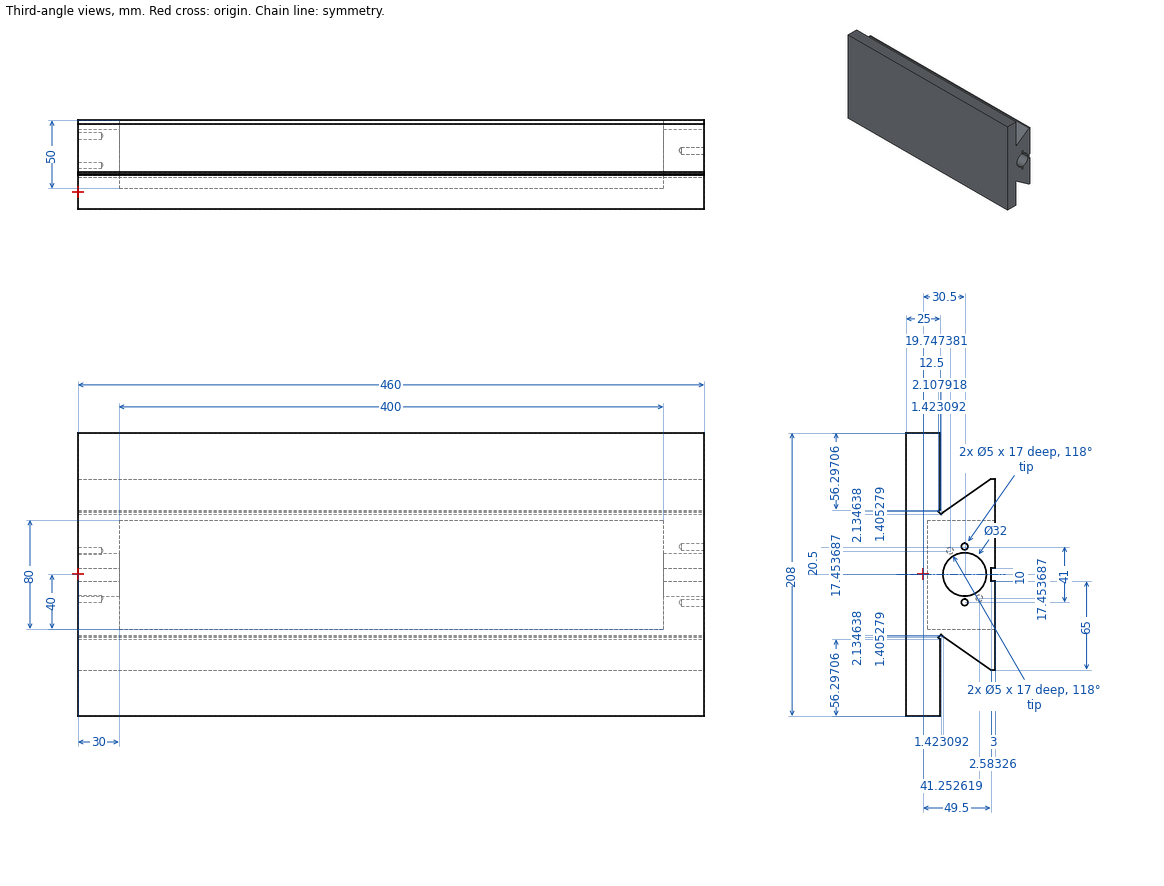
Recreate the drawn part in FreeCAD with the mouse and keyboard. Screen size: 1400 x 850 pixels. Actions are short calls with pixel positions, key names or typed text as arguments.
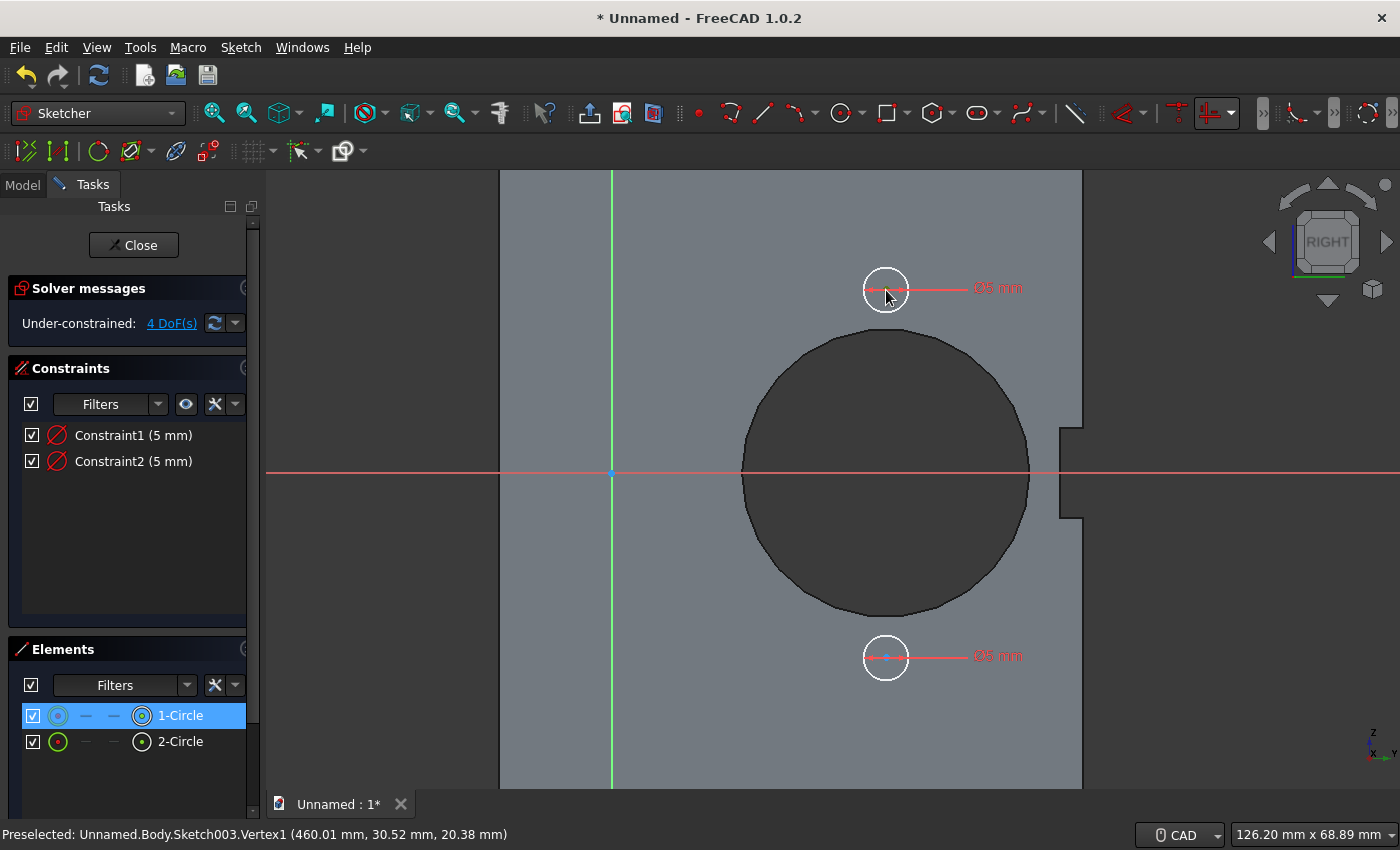
click(886, 658)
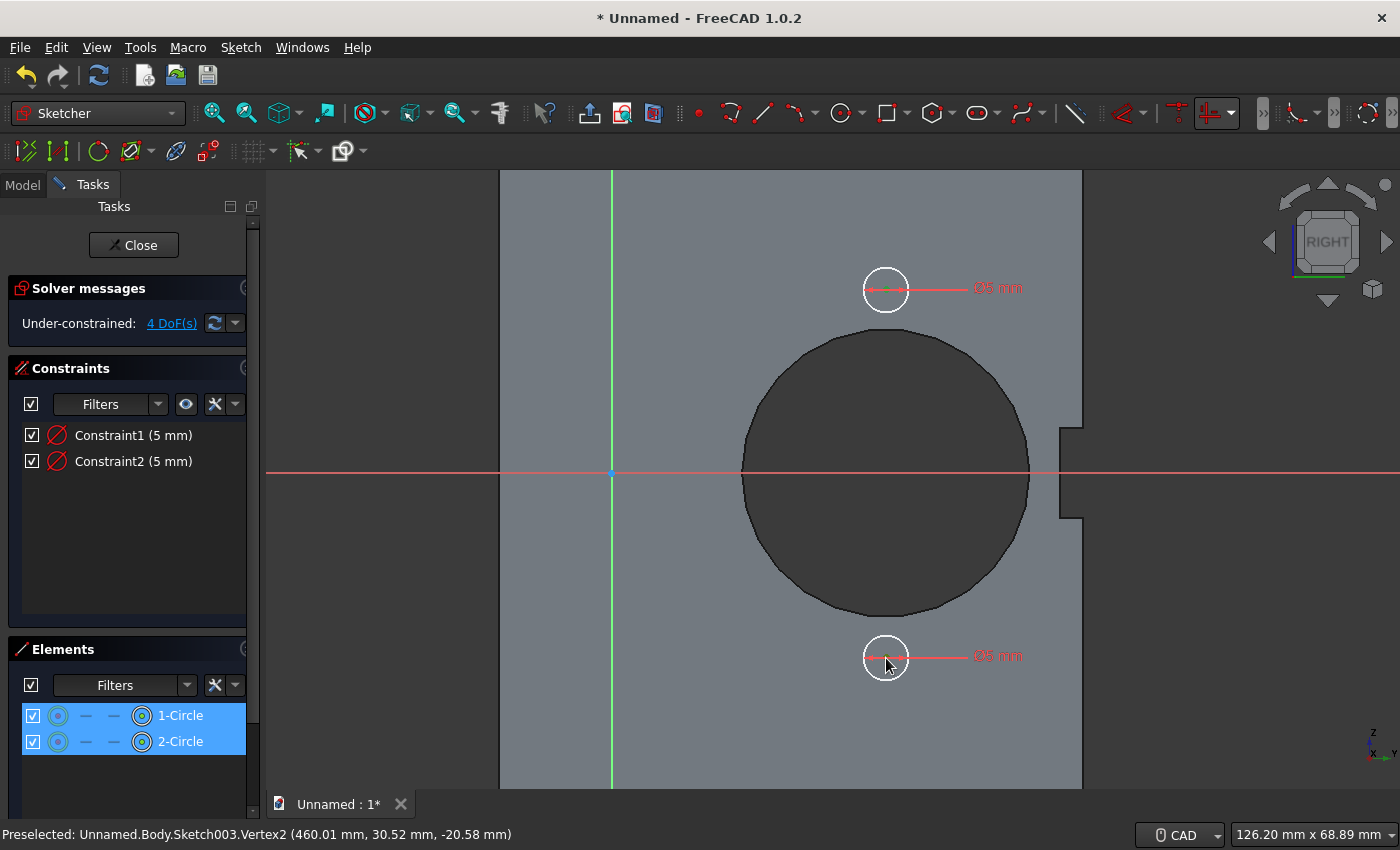
click(1234, 114)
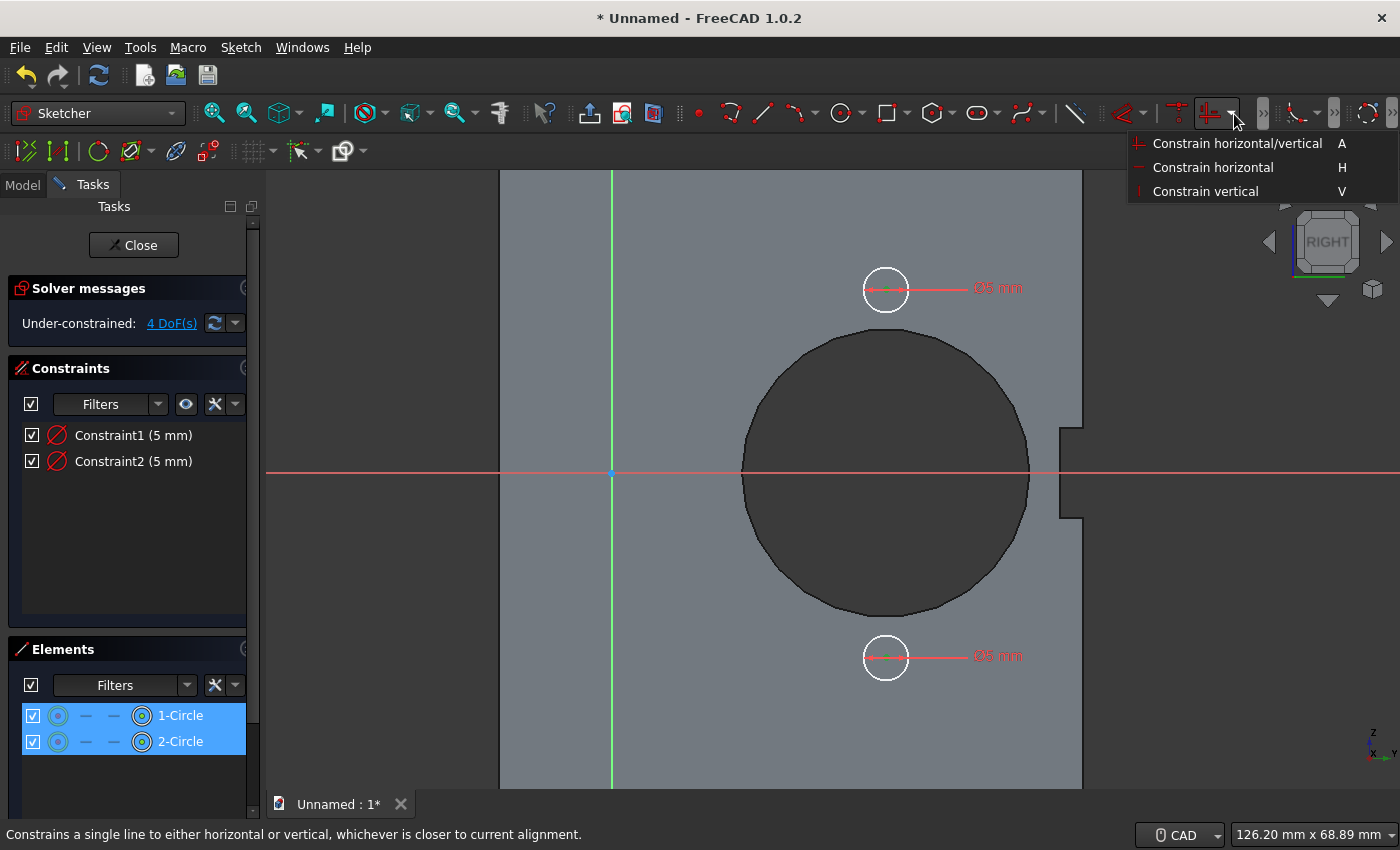
click(1263, 191)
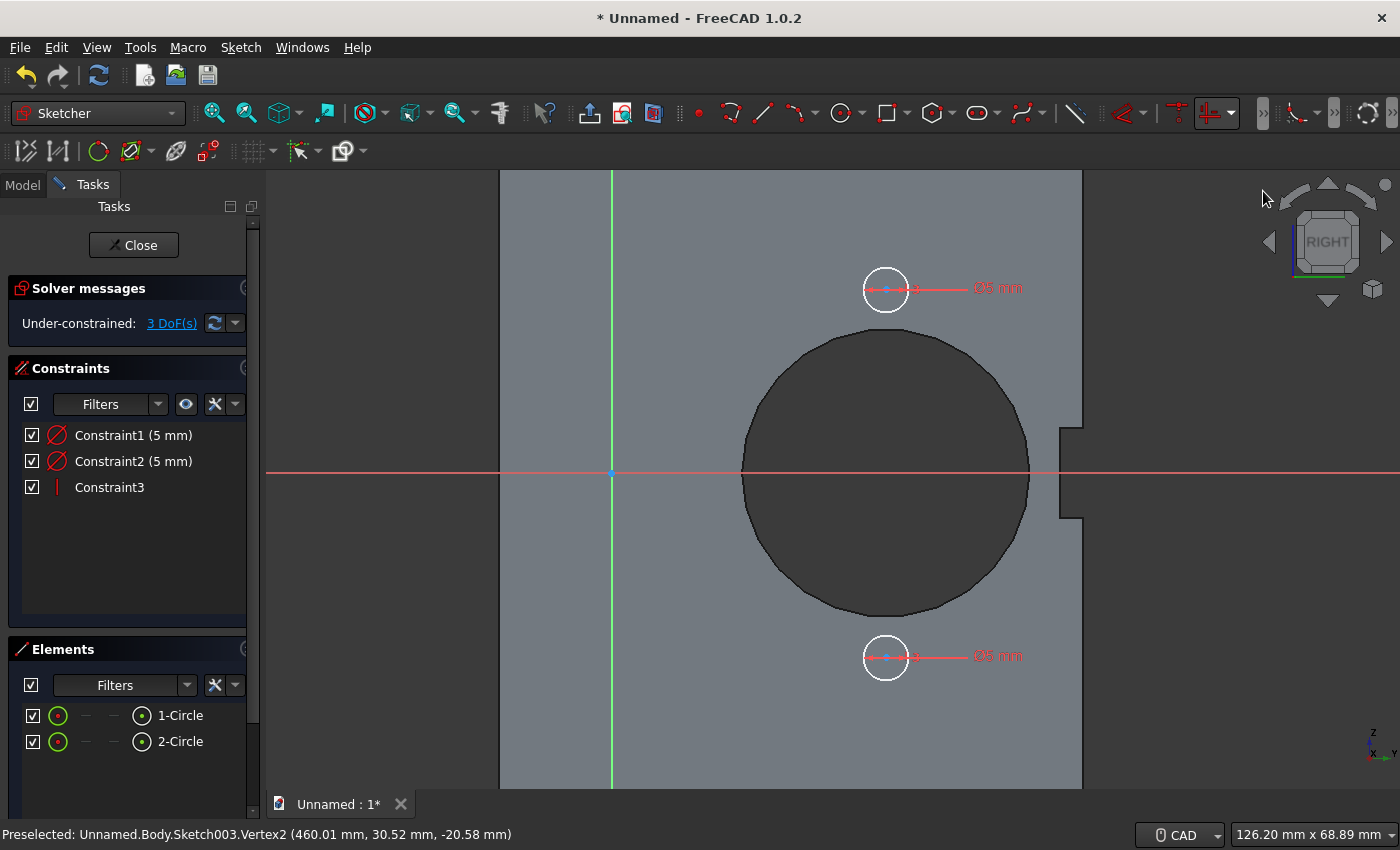
click(1122, 114)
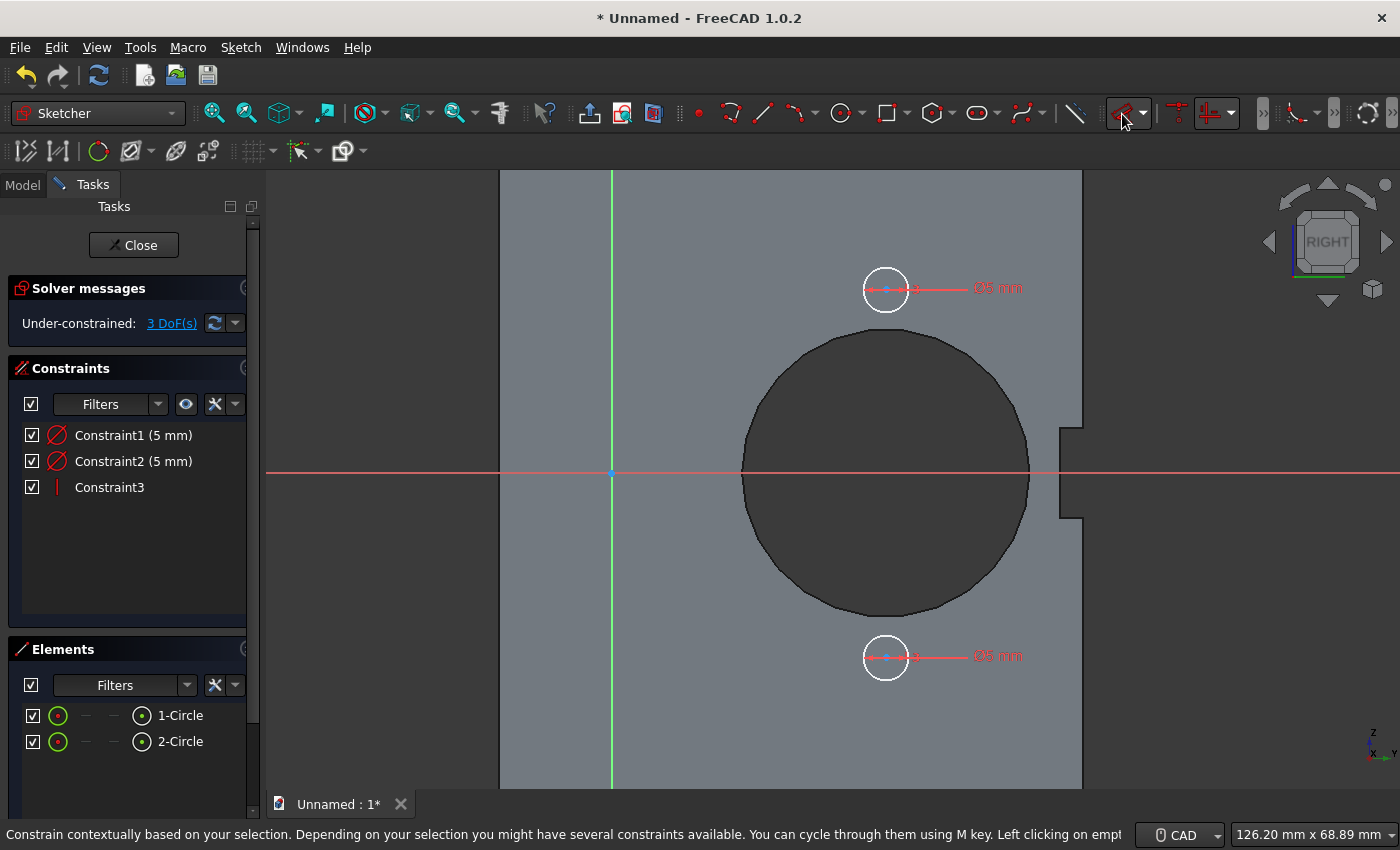
click(886, 290)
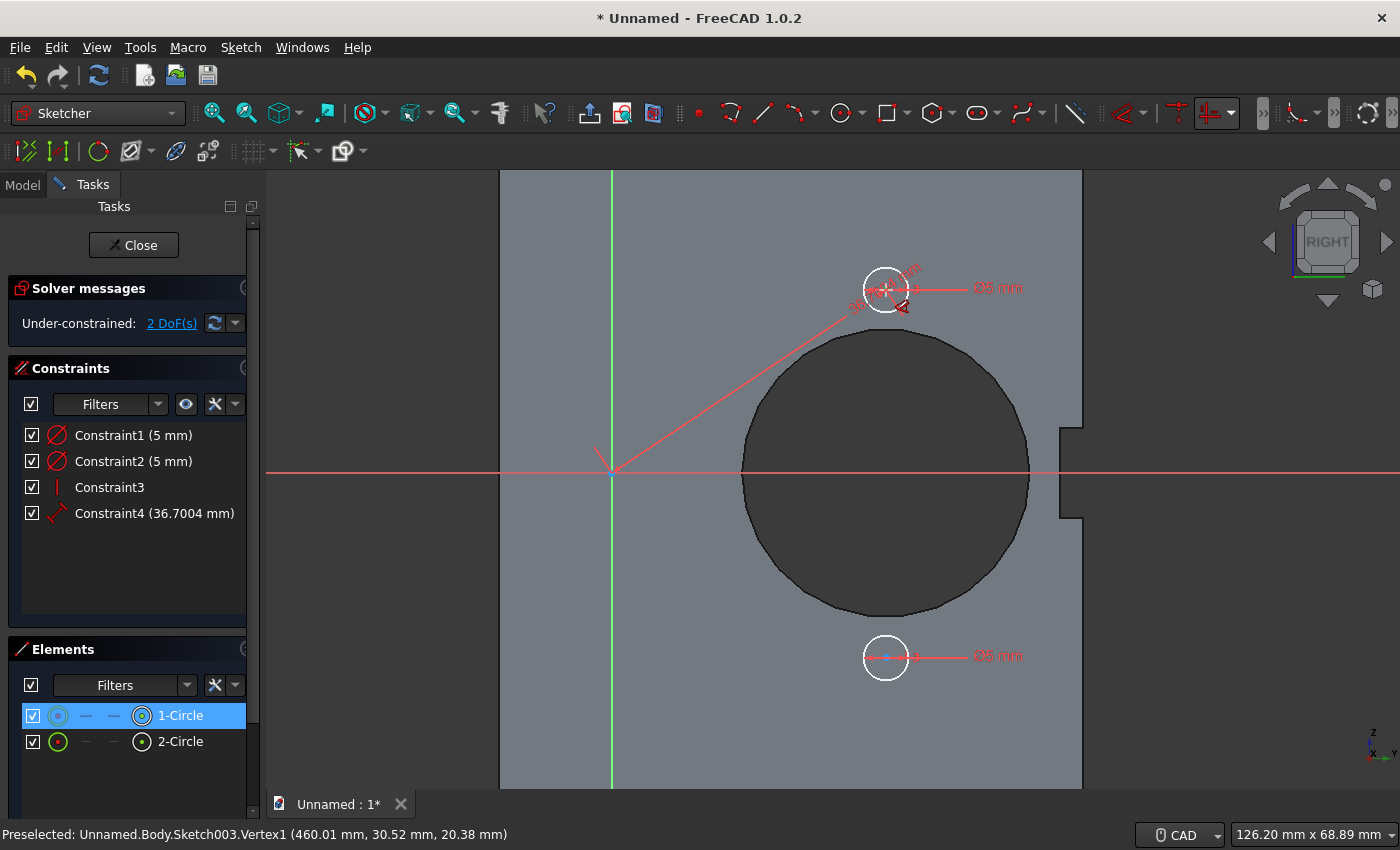
click(886, 658)
click(920, 389)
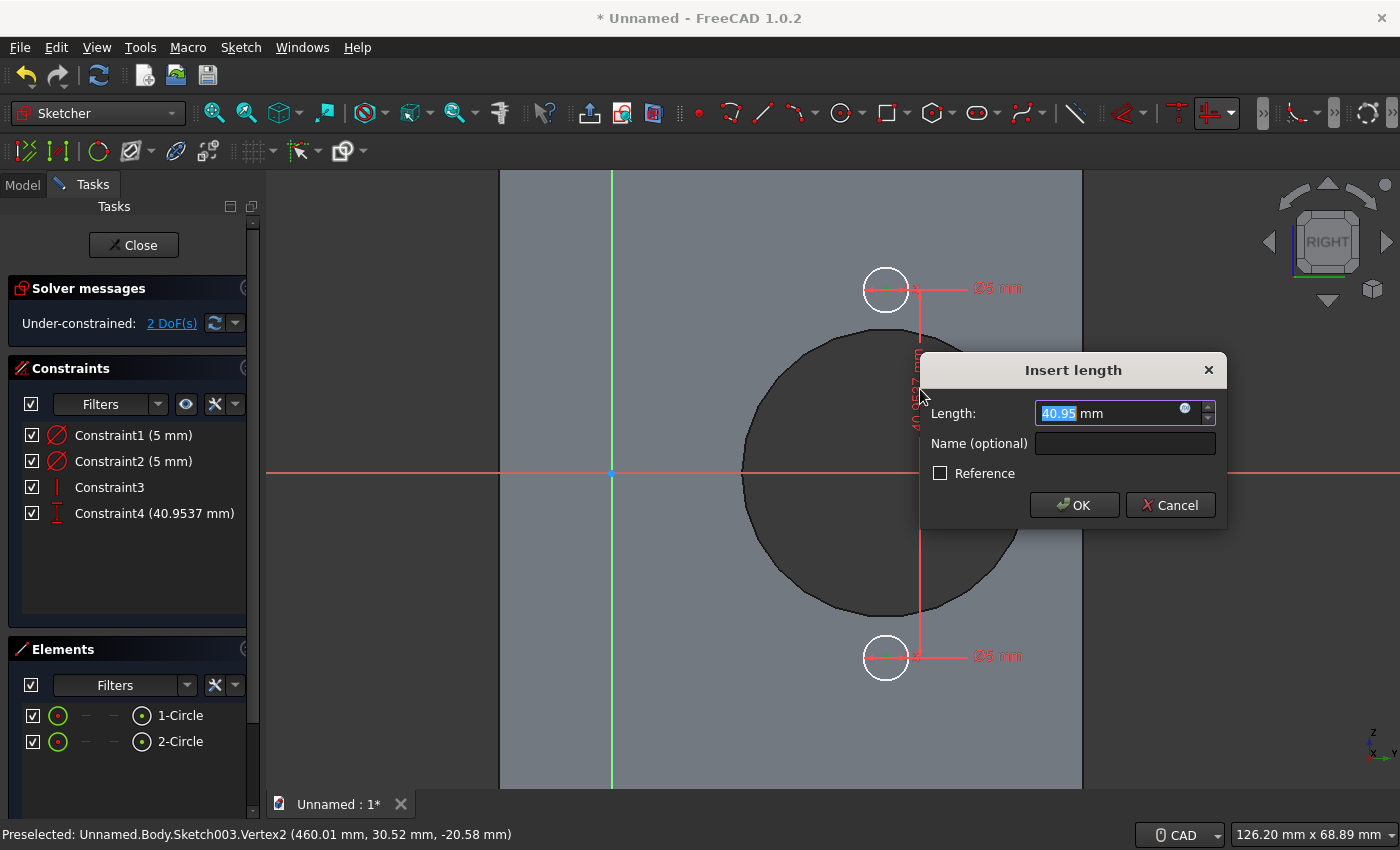
text(41)
key(Return)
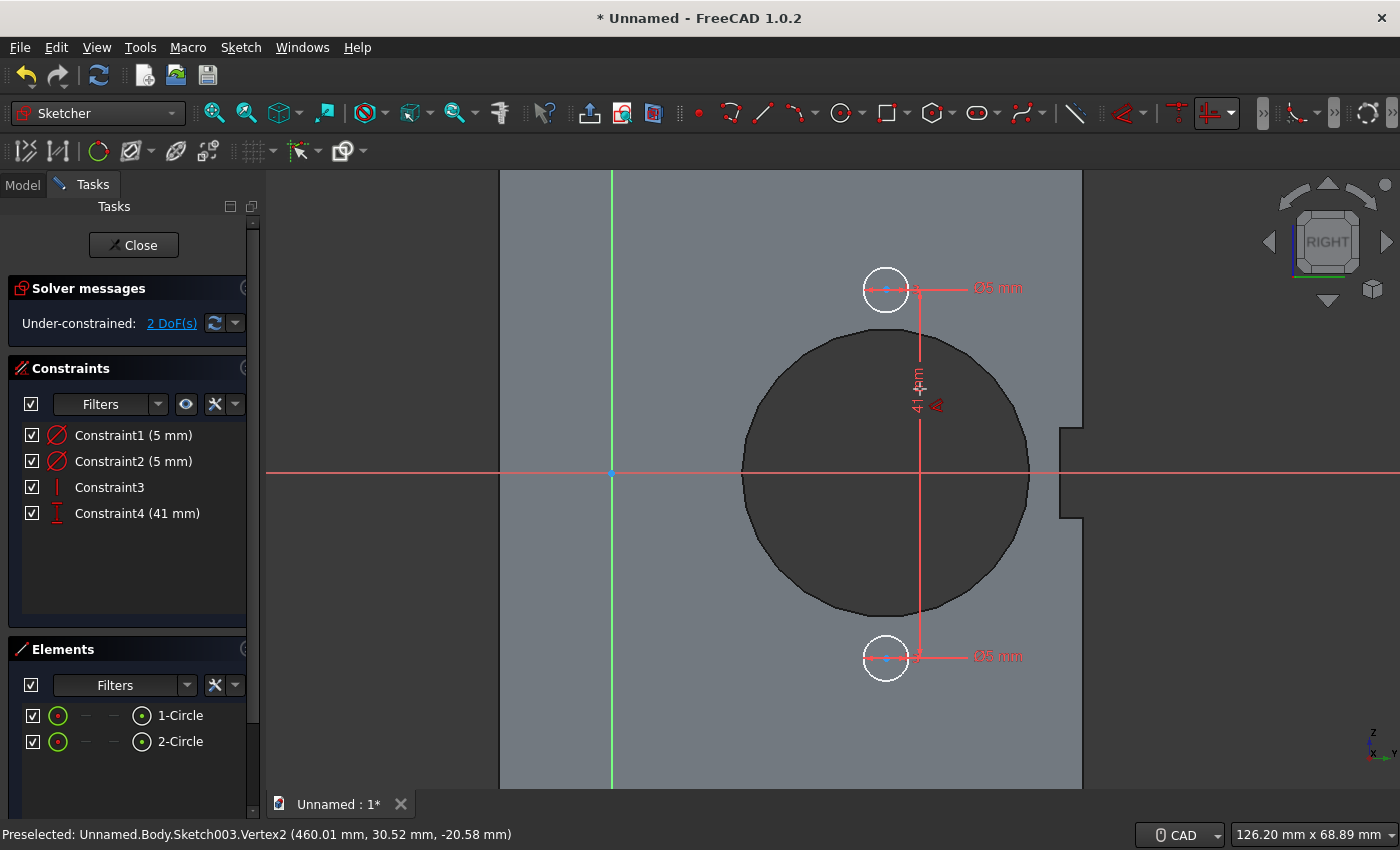
click(886, 290)
click(749, 256)